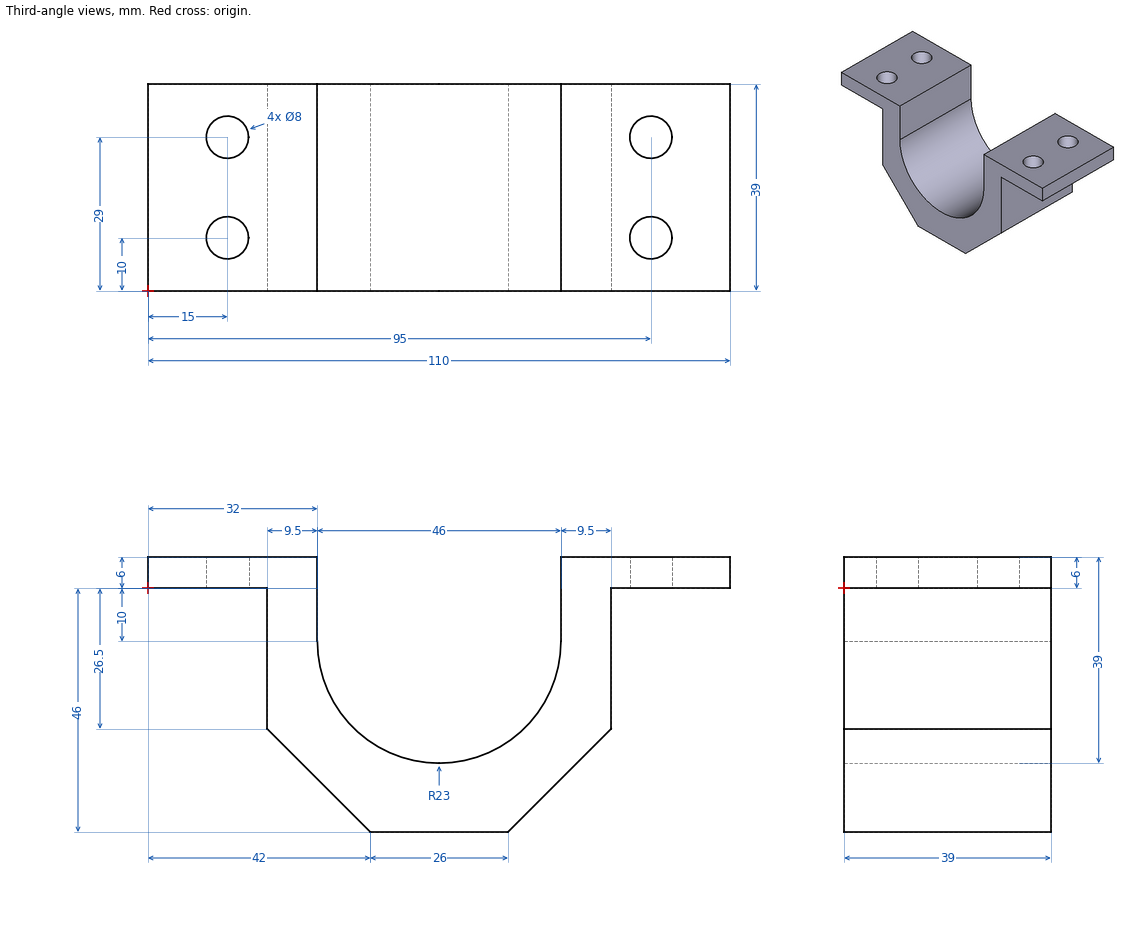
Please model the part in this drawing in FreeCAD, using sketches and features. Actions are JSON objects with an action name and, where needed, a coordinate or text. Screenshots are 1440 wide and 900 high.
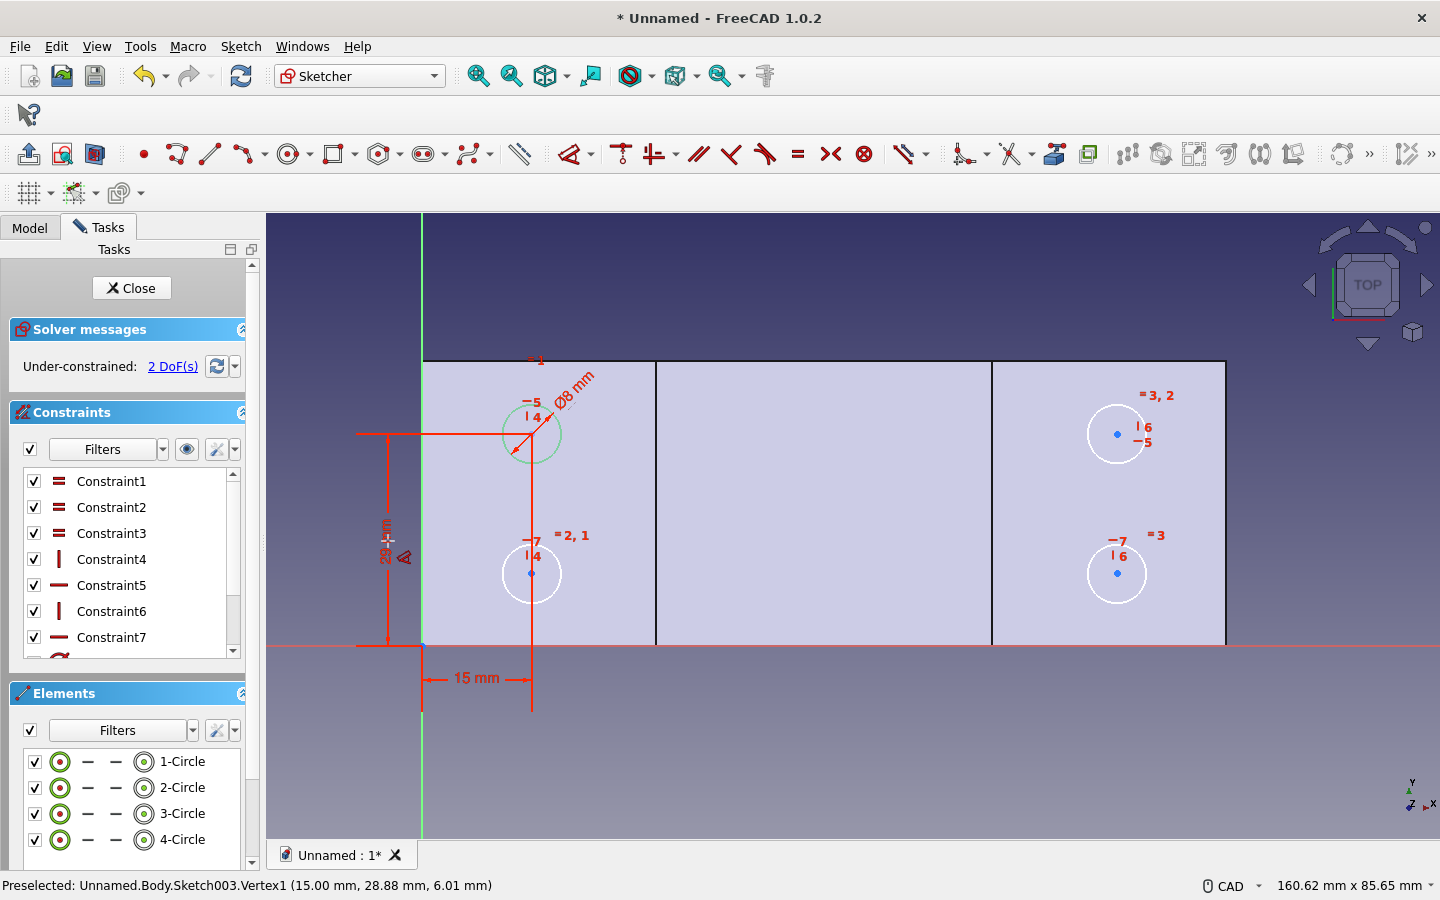
{"action": "left_click", "coordinate": [532, 574]}
{"action": "left_click", "coordinate": [388, 610]}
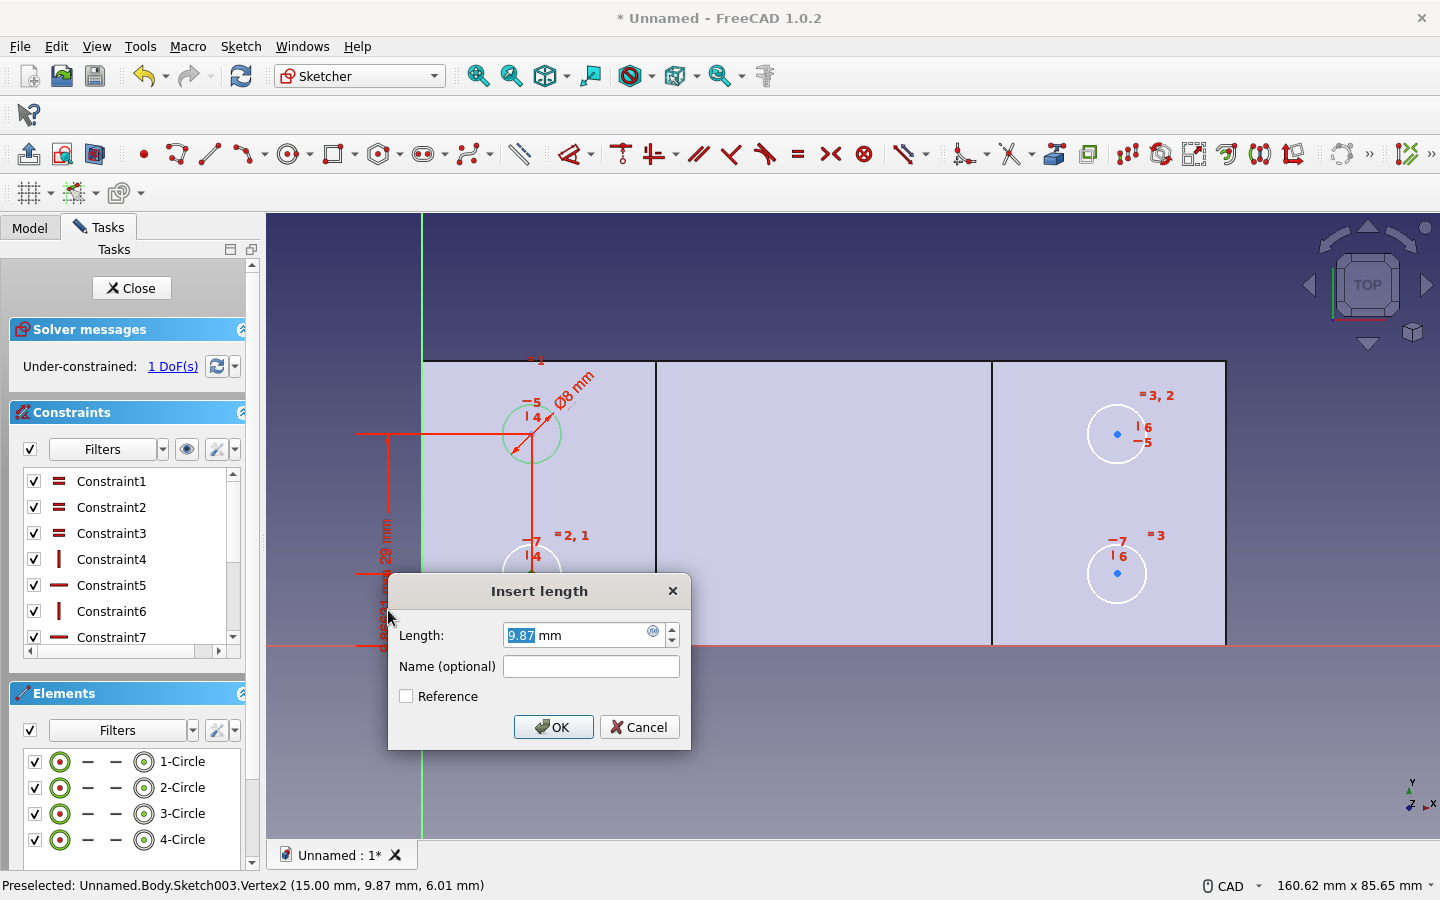
{"action": "type", "text": "10"}
{"action": "key", "text": "Return"}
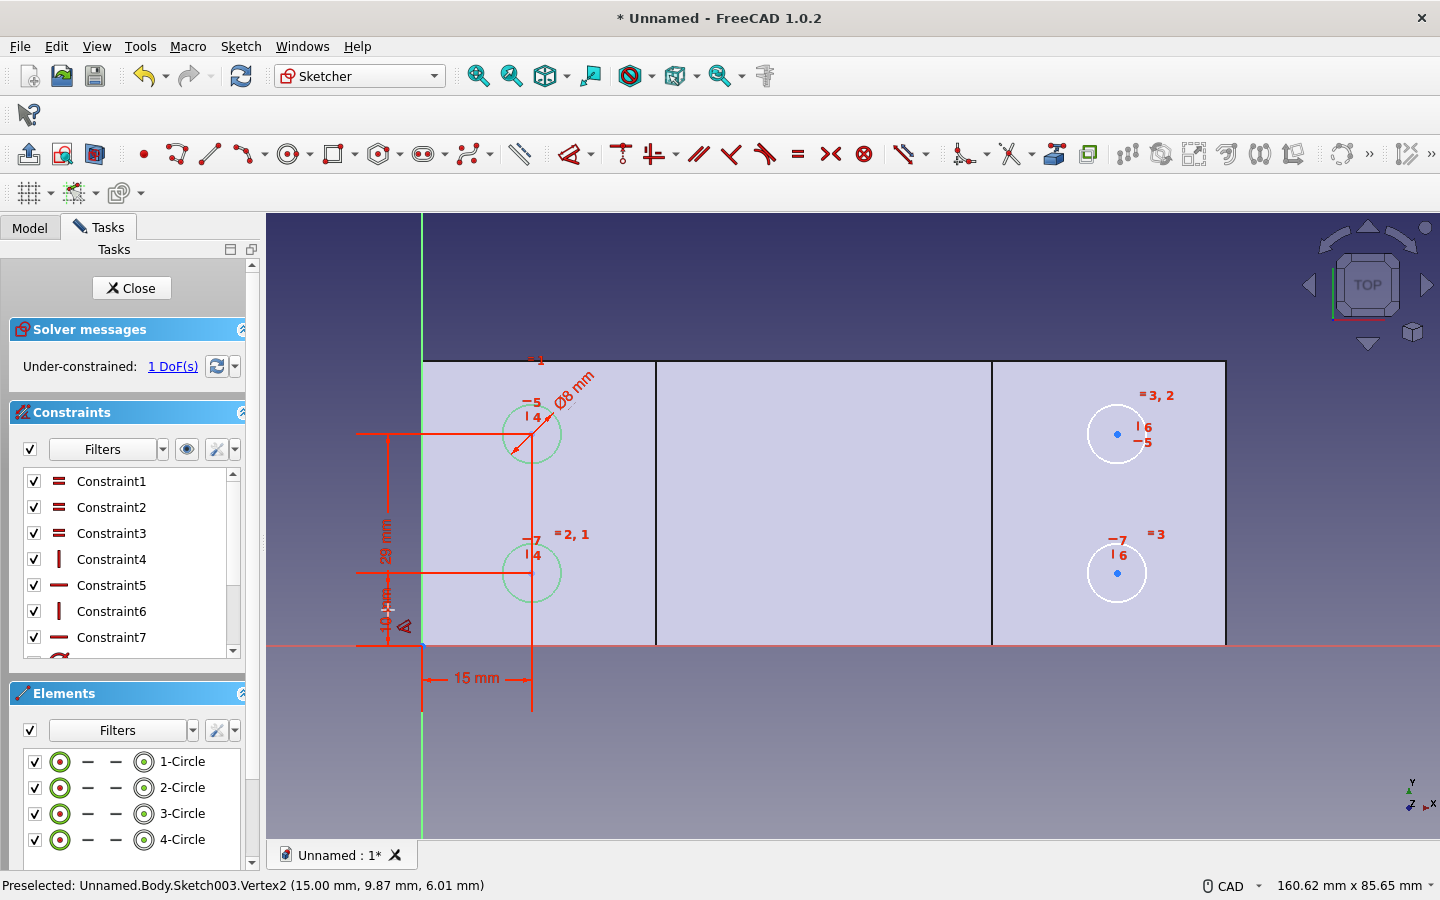
{"action": "left_click", "coordinate": [1117, 434]}
{"action": "left_click", "coordinate": [770, 680]}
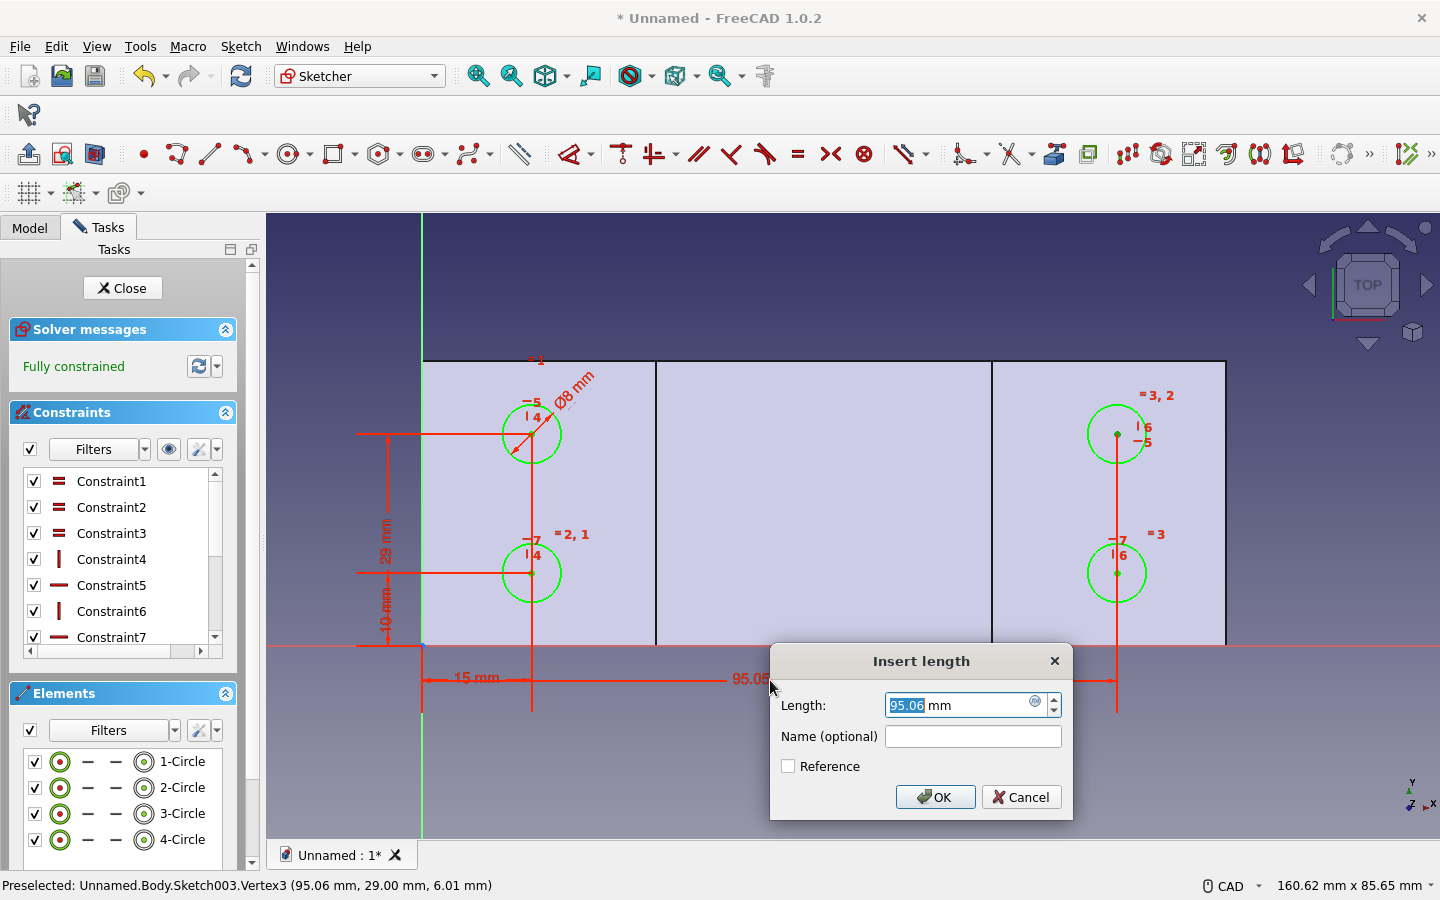
{"action": "type", "text": "95"}
{"action": "key", "text": "Return"}
{"action": "key", "text": "Escape"}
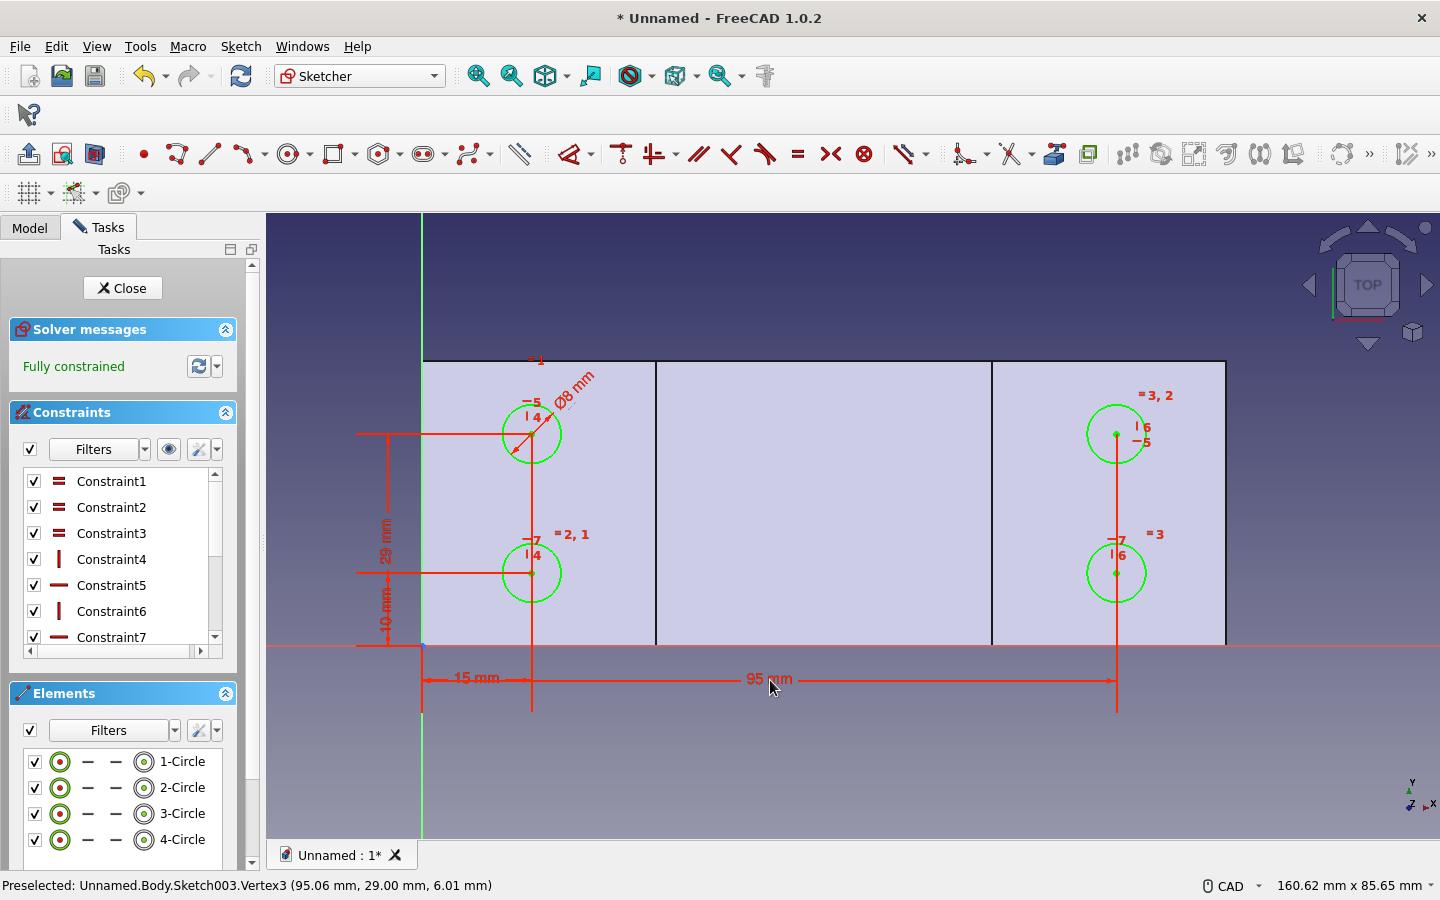
{"action": "left_click", "coordinate": [123, 288]}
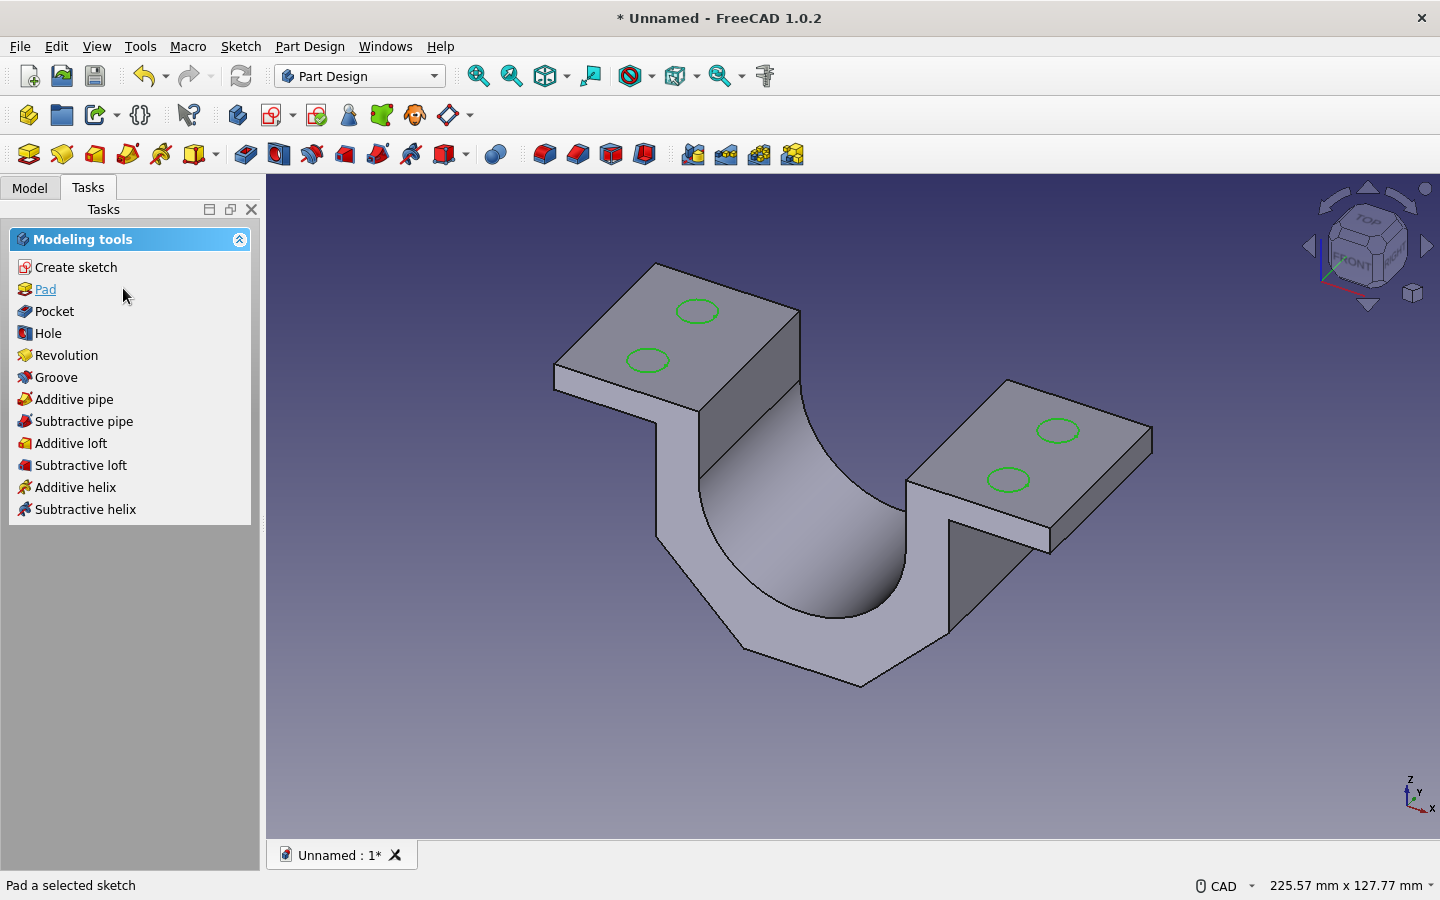
{"action": "left_click", "coordinate": [246, 154]}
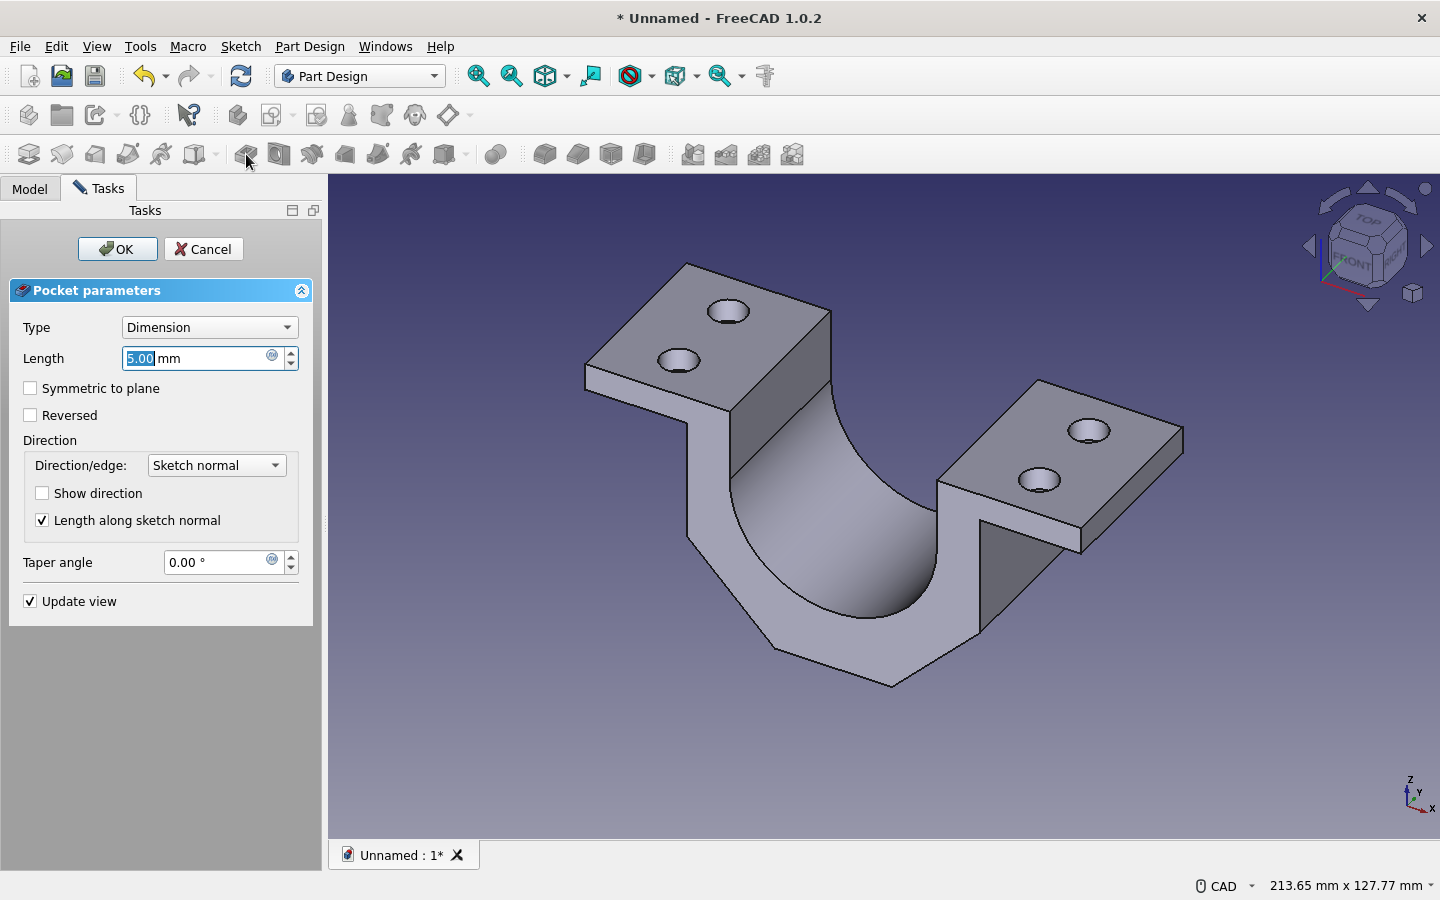
{"action": "type", "text": "39"}
{"action": "key", "text": "Tab"}